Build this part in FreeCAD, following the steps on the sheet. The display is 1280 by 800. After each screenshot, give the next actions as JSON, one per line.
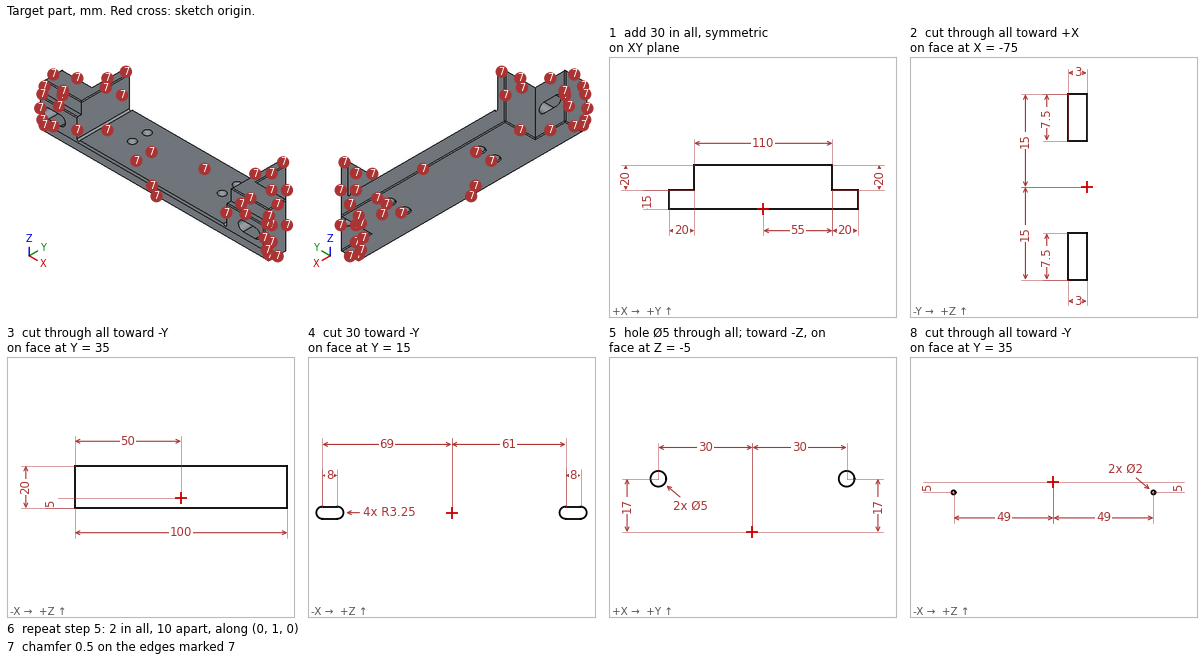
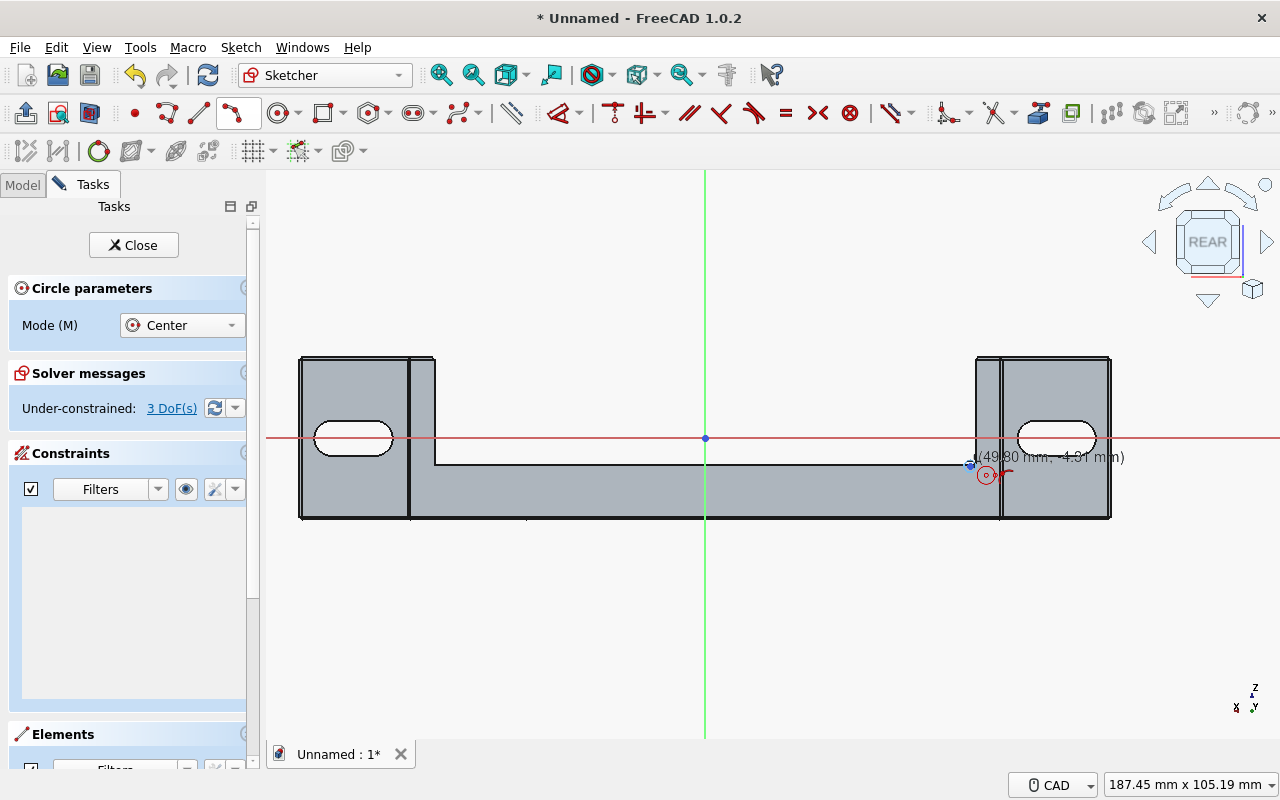
{"action": "scroll", "coordinate": [440, 465], "scroll_direction": "up", "scroll_amount": 8}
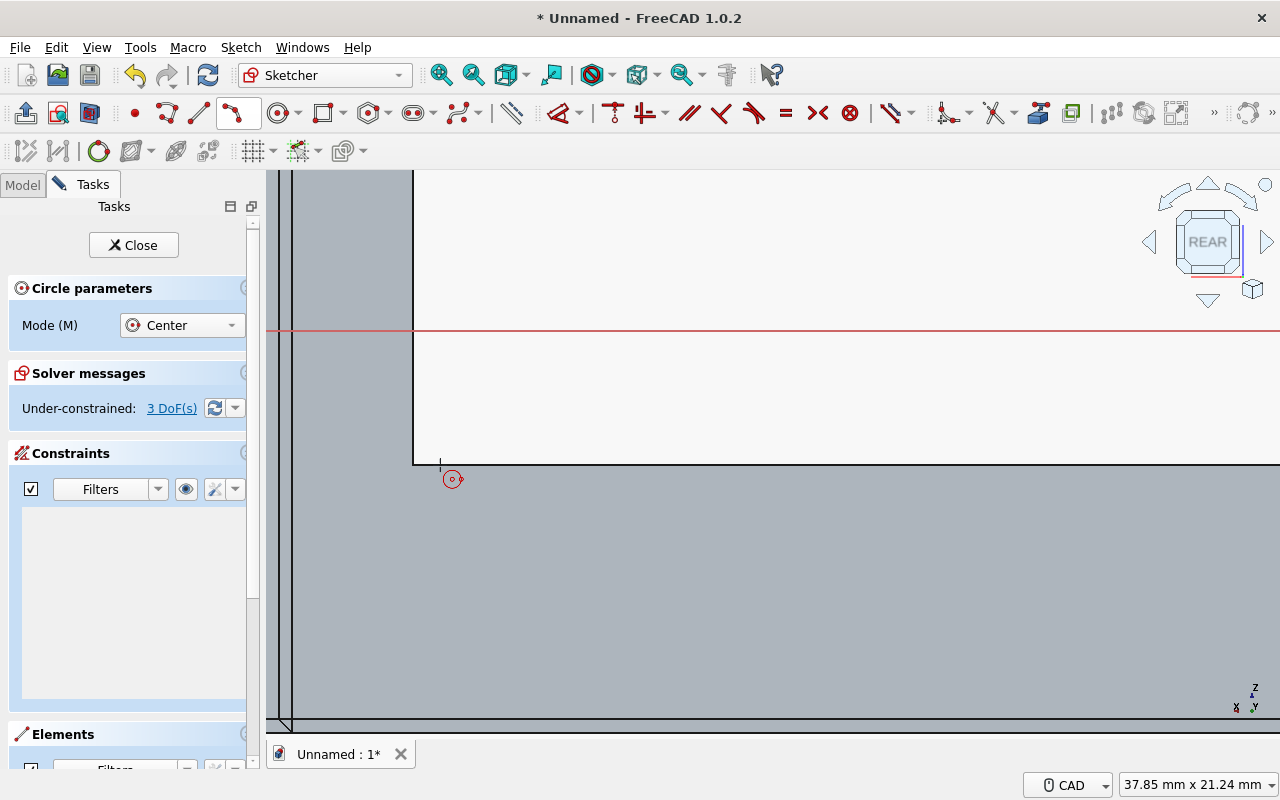
{"action": "scroll", "coordinate": [439, 465], "scroll_direction": "down", "scroll_amount": 8}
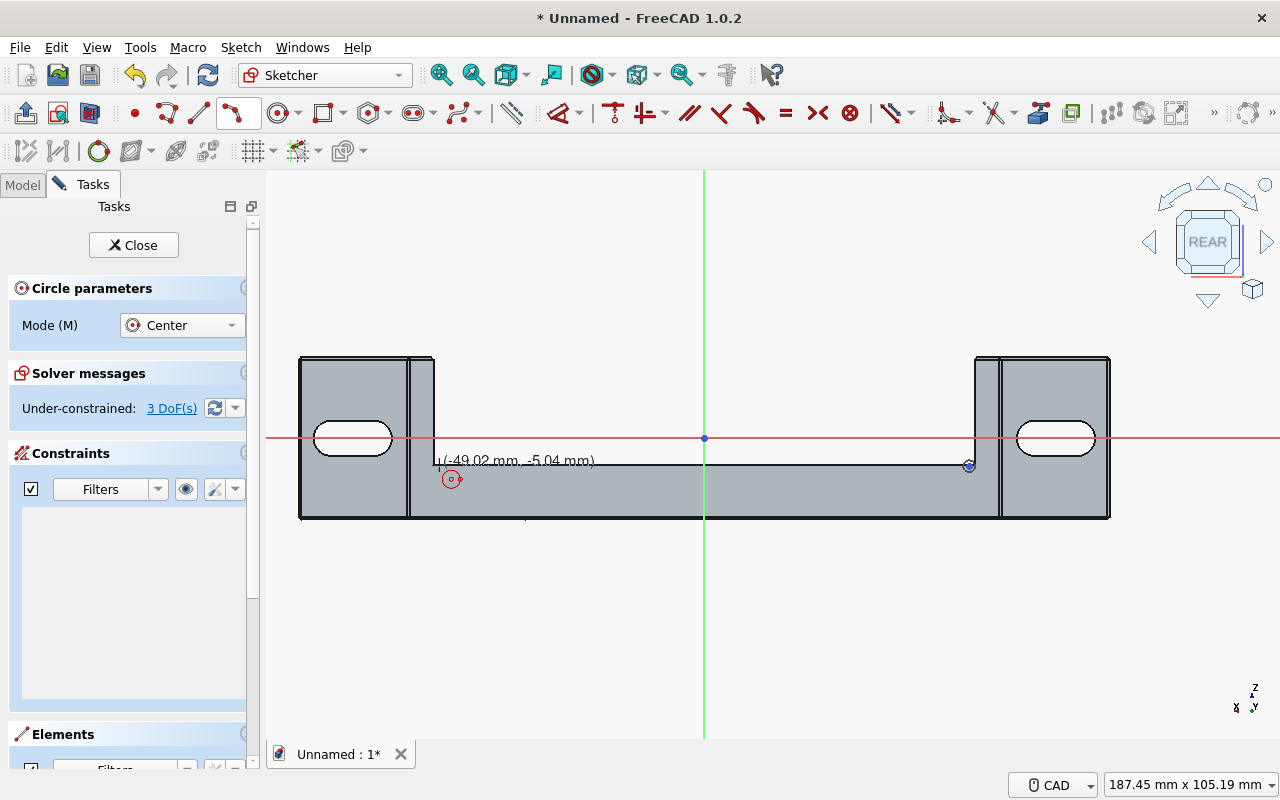
{"action": "left_click", "coordinate": [439, 465]}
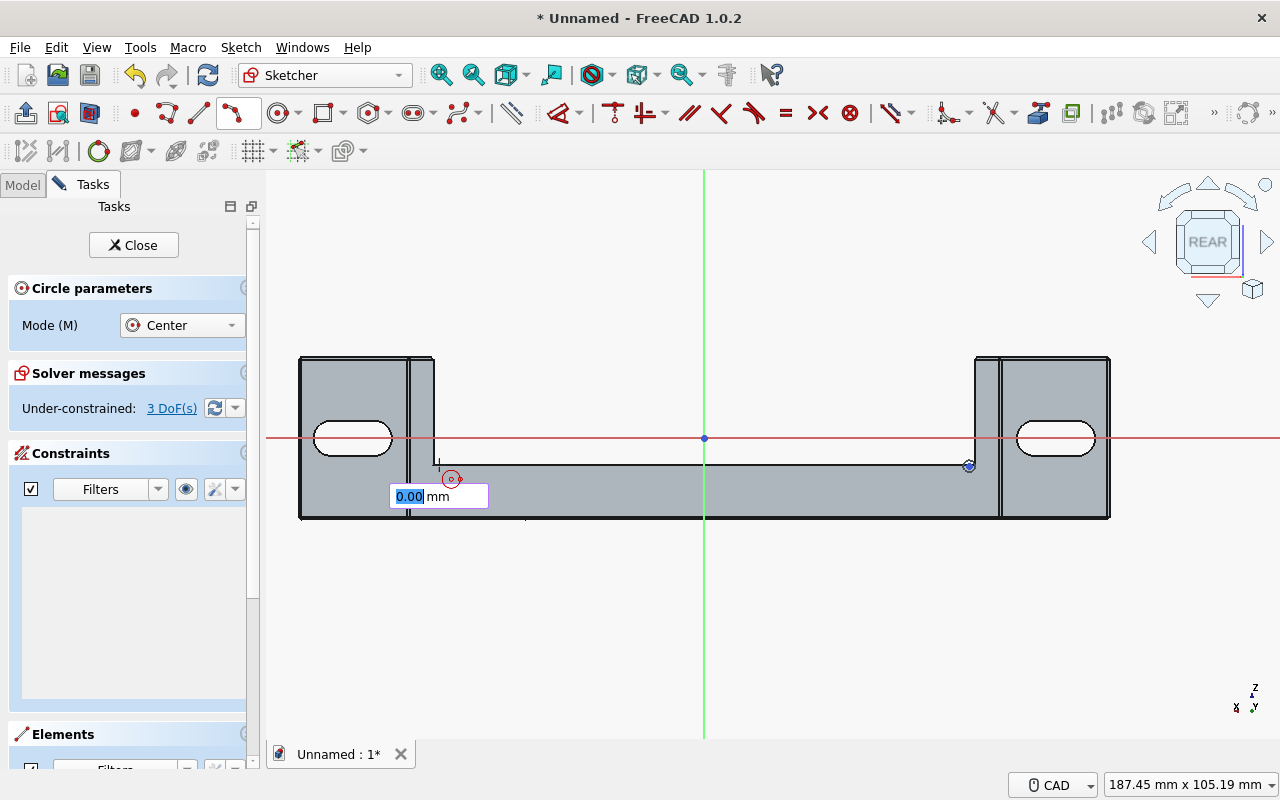
{"action": "scroll", "coordinate": [443, 462], "scroll_direction": "up", "scroll_amount": 6}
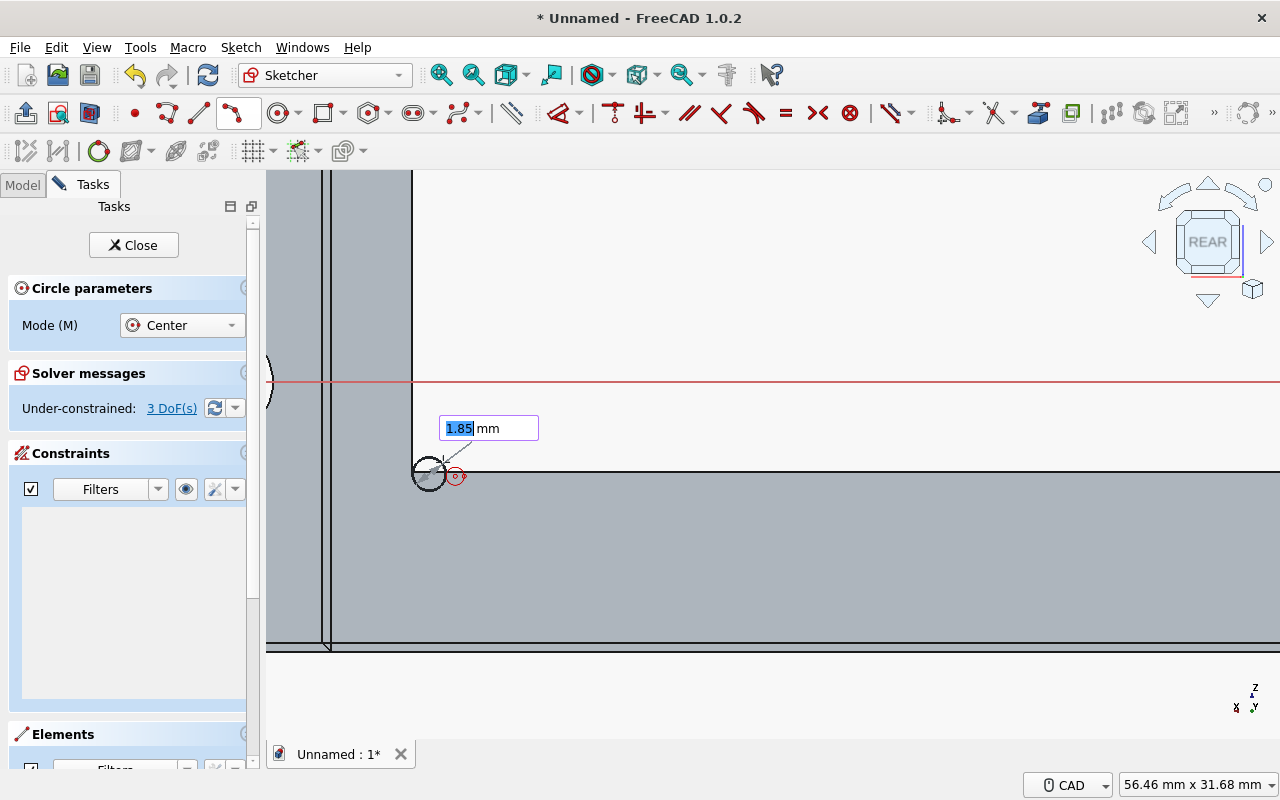
{"action": "left_click", "coordinate": [443, 459]}
{"action": "key", "text": "Escape"}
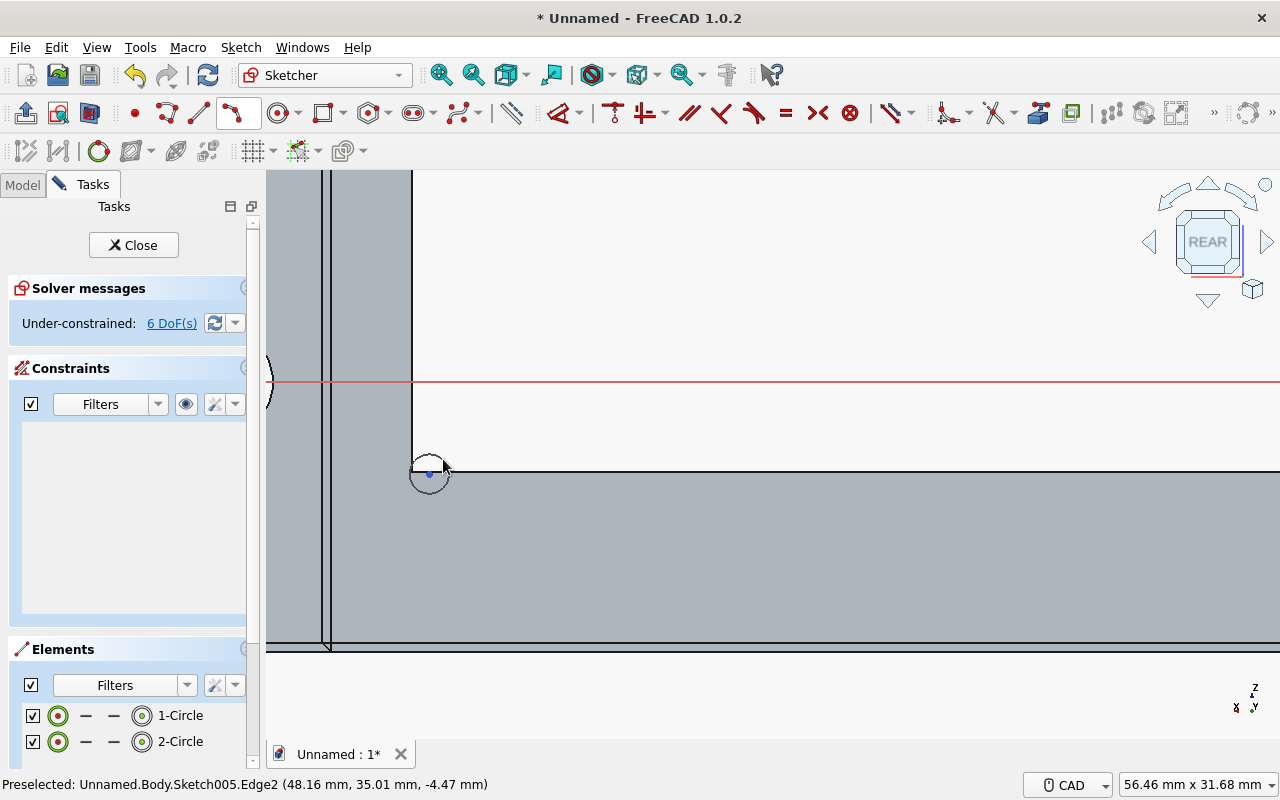
{"action": "scroll", "coordinate": [443, 462], "scroll_direction": "down", "scroll_amount": 6}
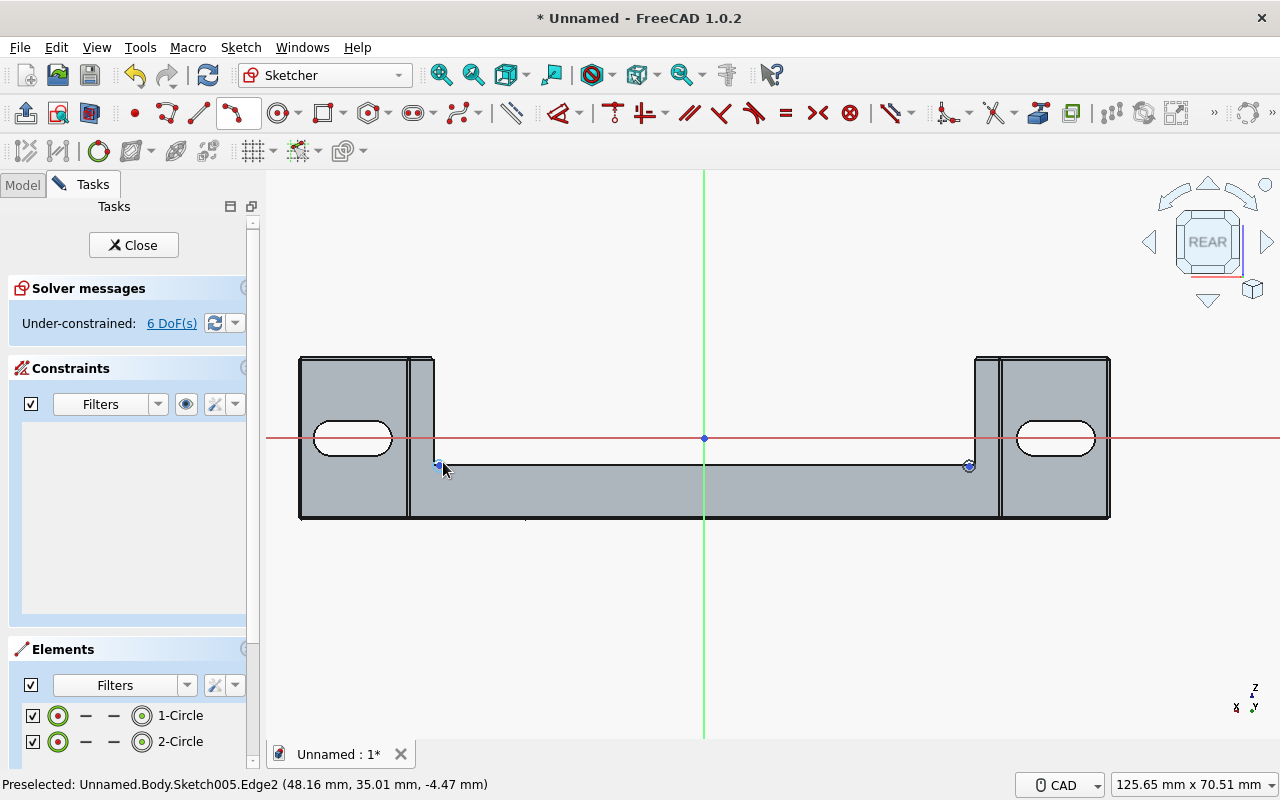
{"action": "scroll", "coordinate": [973, 462], "scroll_direction": "up", "scroll_amount": 5}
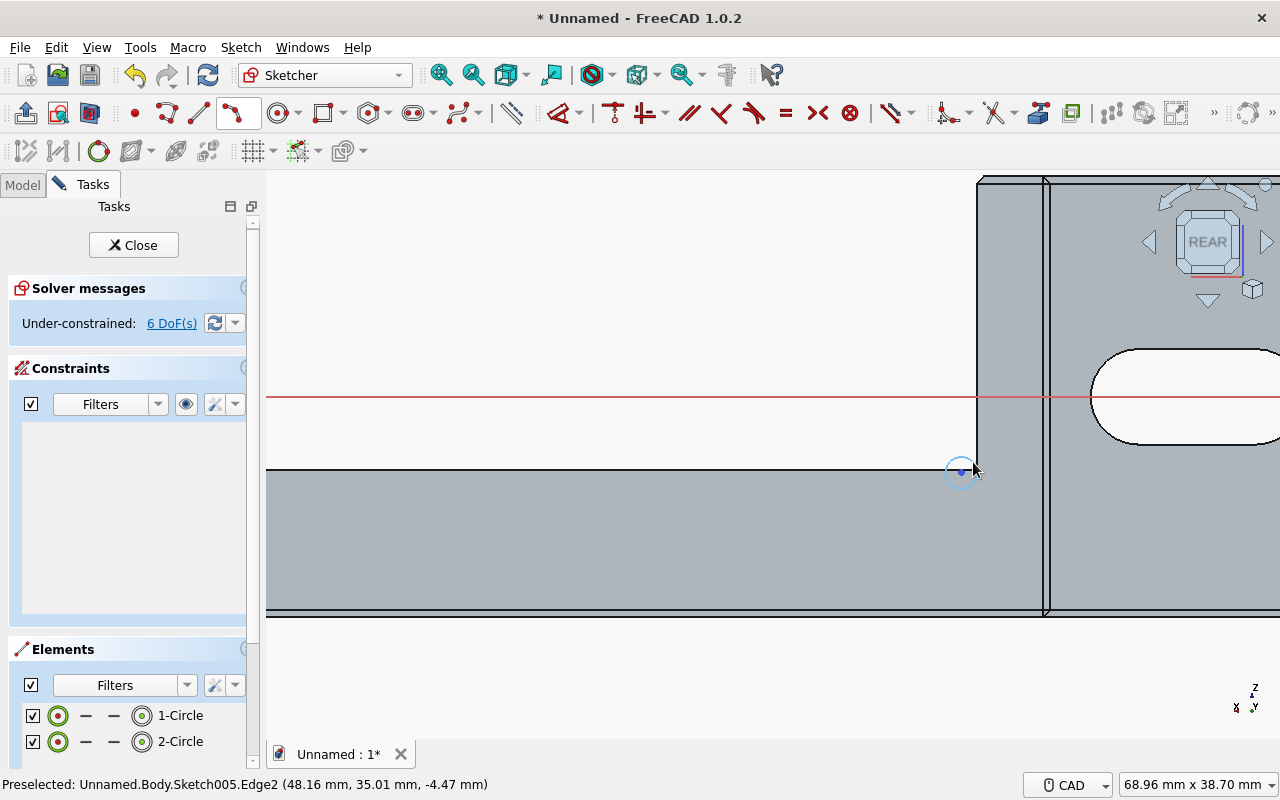
{"action": "left_click", "coordinate": [973, 462]}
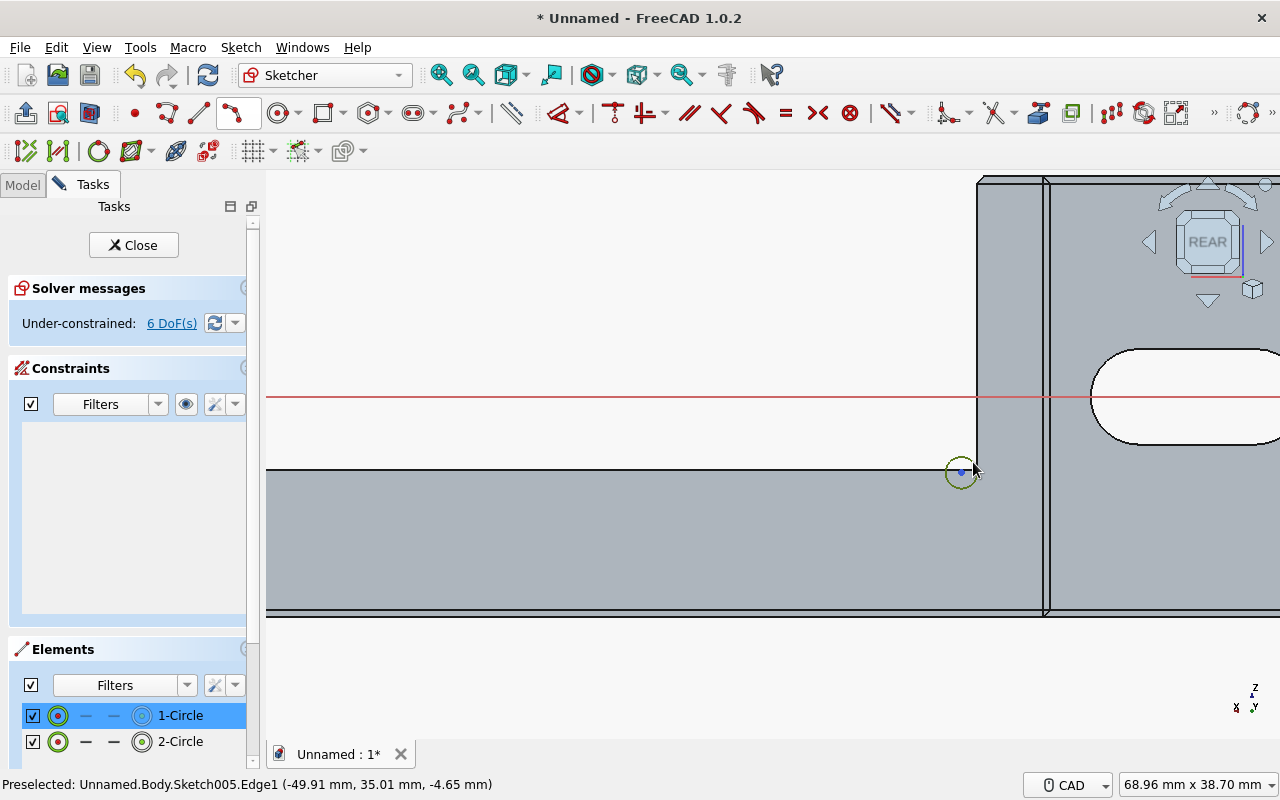
{"action": "scroll", "coordinate": [974, 462], "scroll_direction": "down", "scroll_amount": 5}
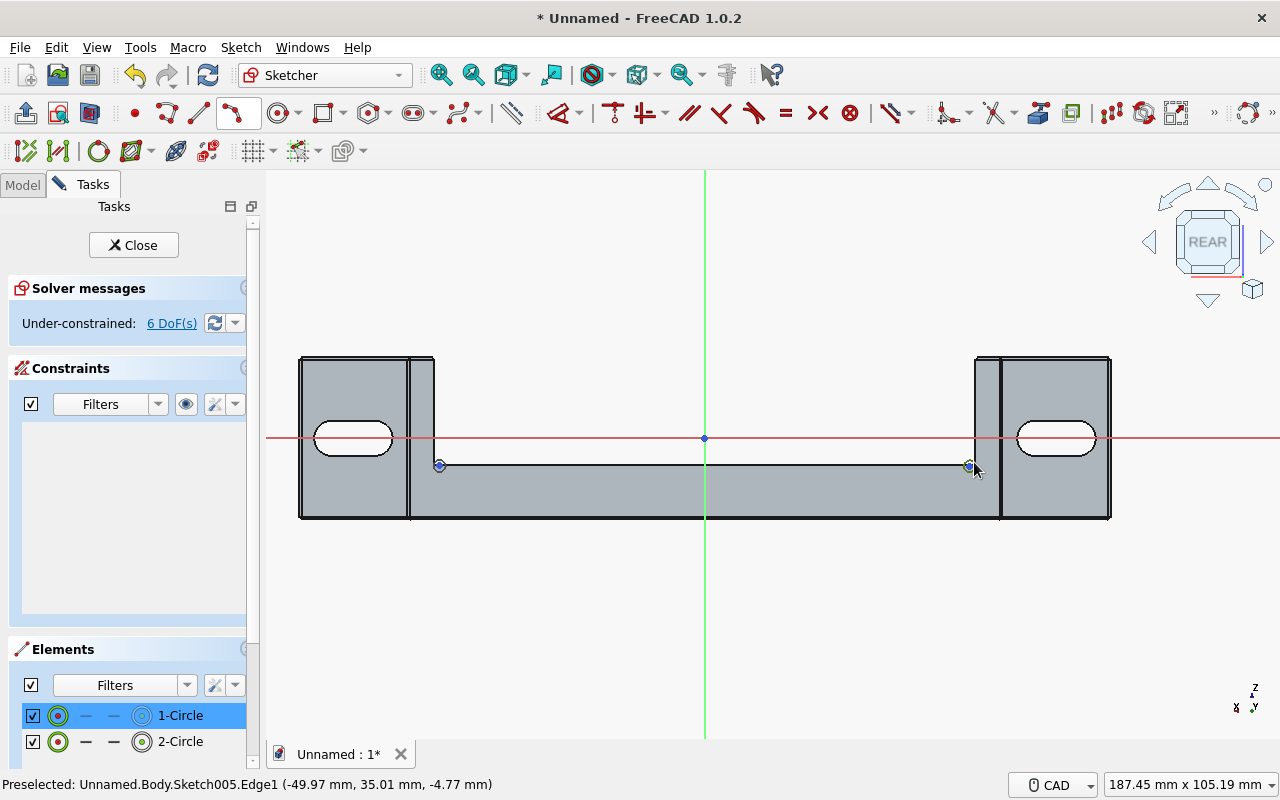
{"action": "scroll", "coordinate": [444, 462], "scroll_direction": "up", "scroll_amount": 5}